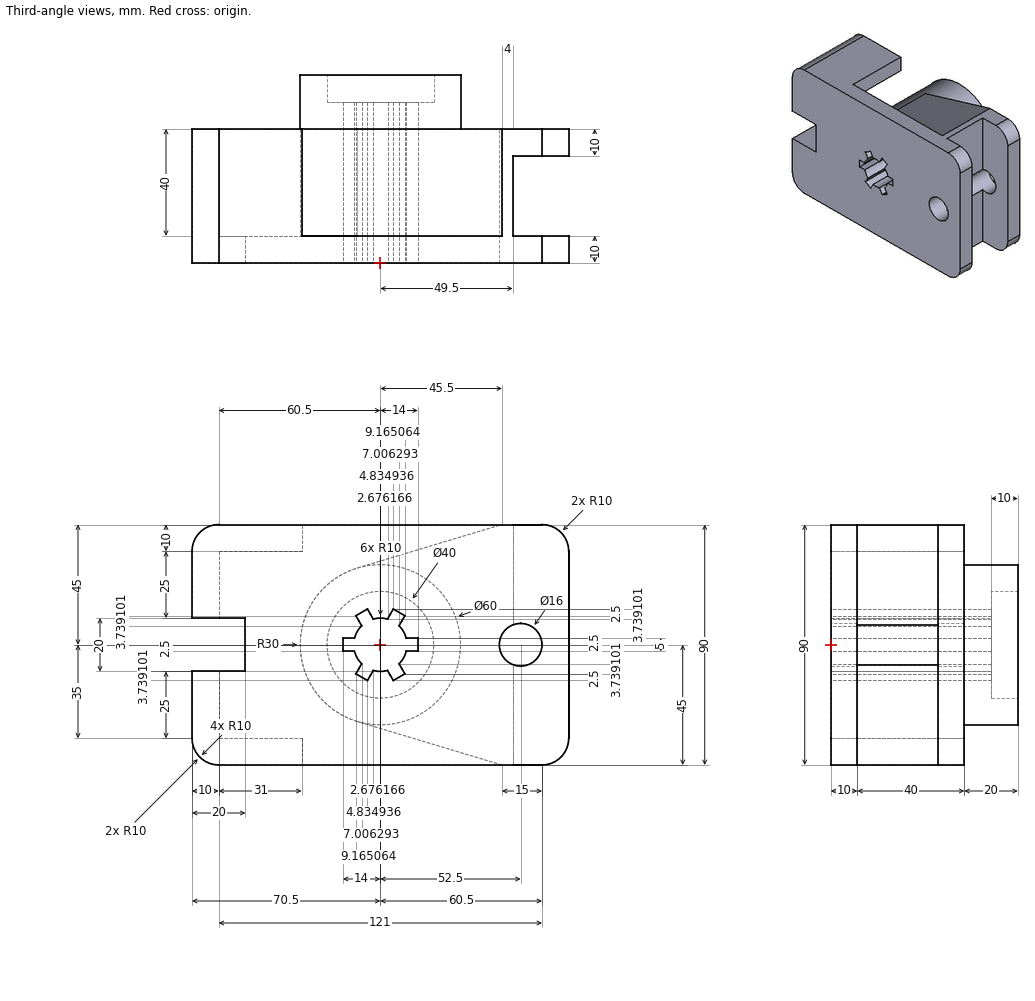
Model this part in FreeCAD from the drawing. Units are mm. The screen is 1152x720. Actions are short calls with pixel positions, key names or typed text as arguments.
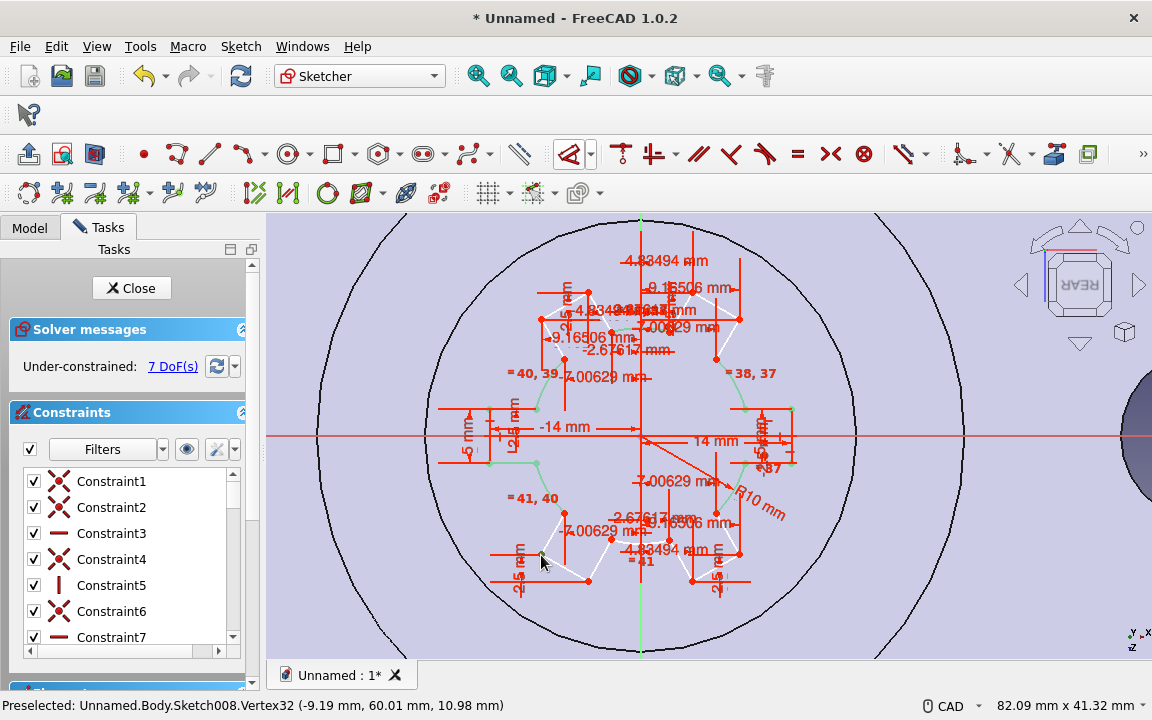
click(590, 154)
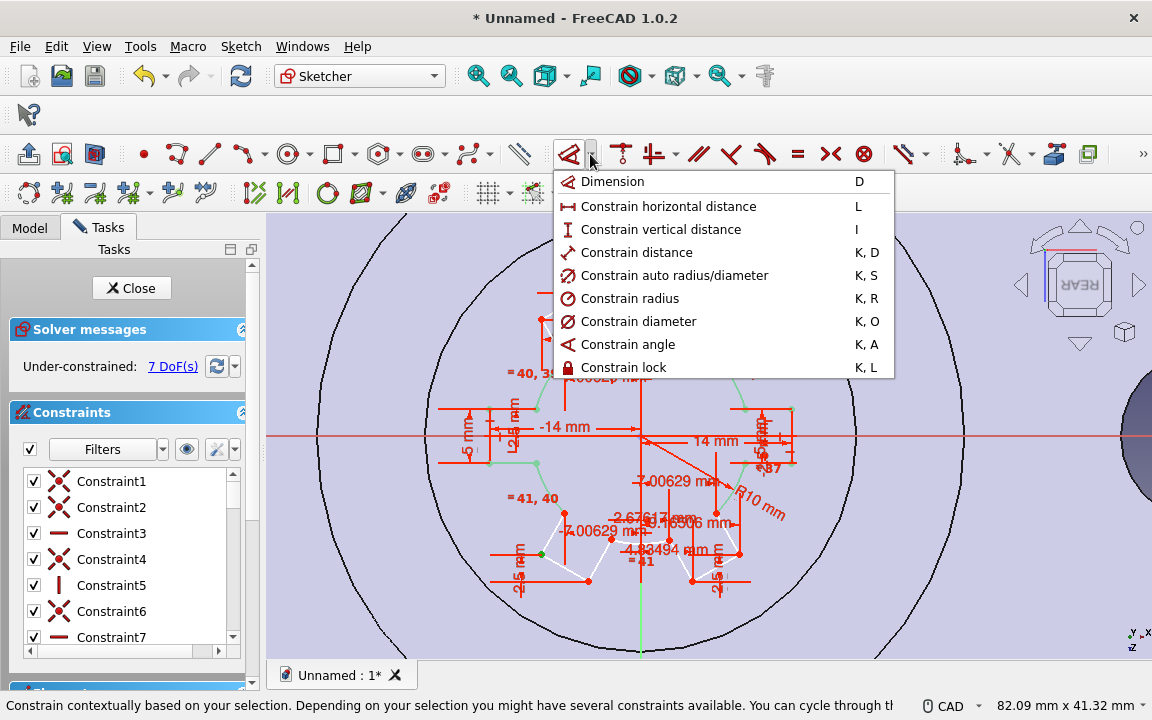
click(724, 206)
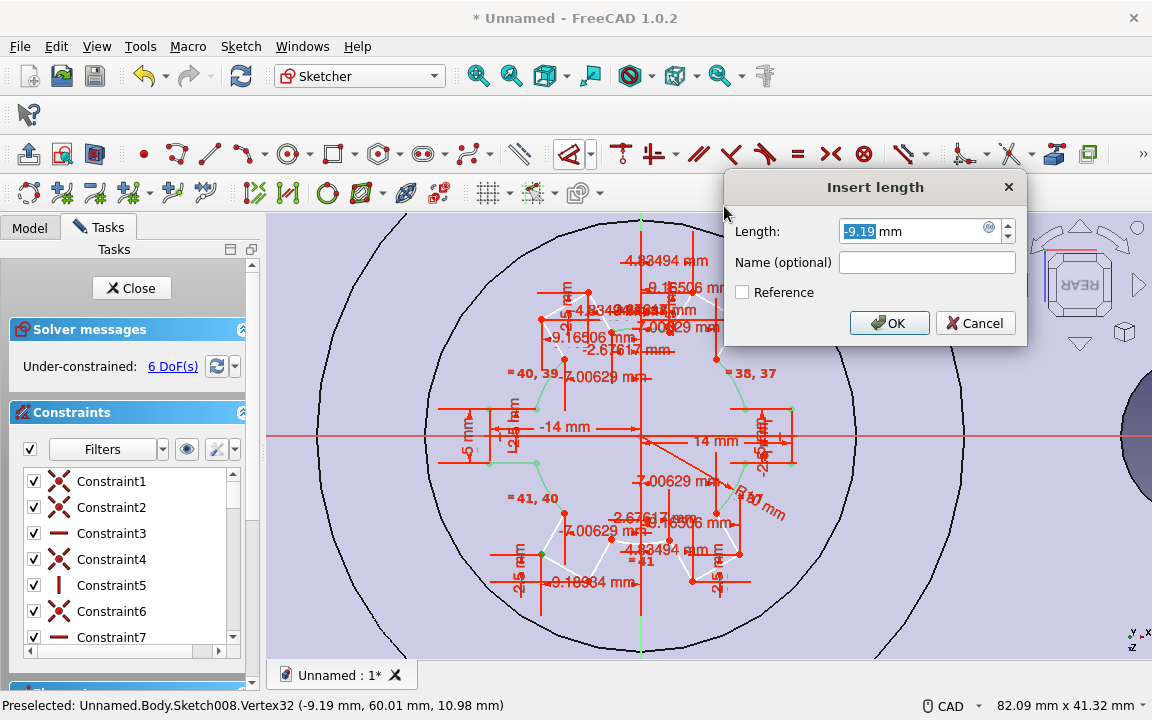
text(-9.165064)
key(Return)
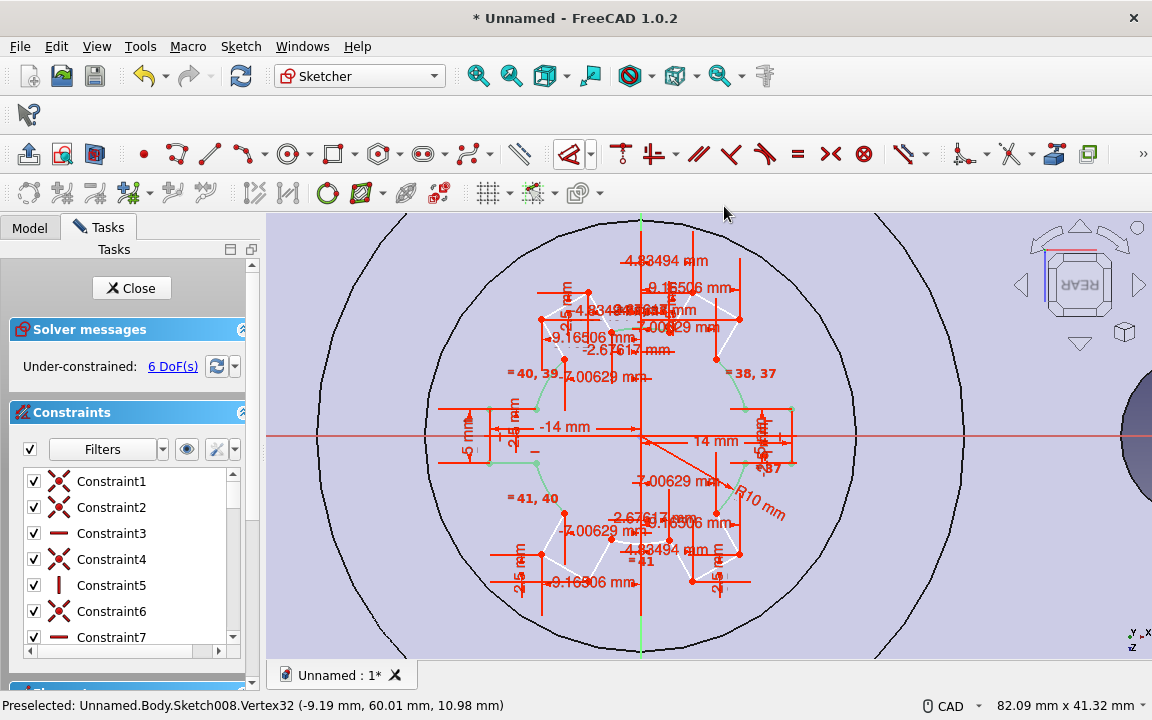
click(588, 582)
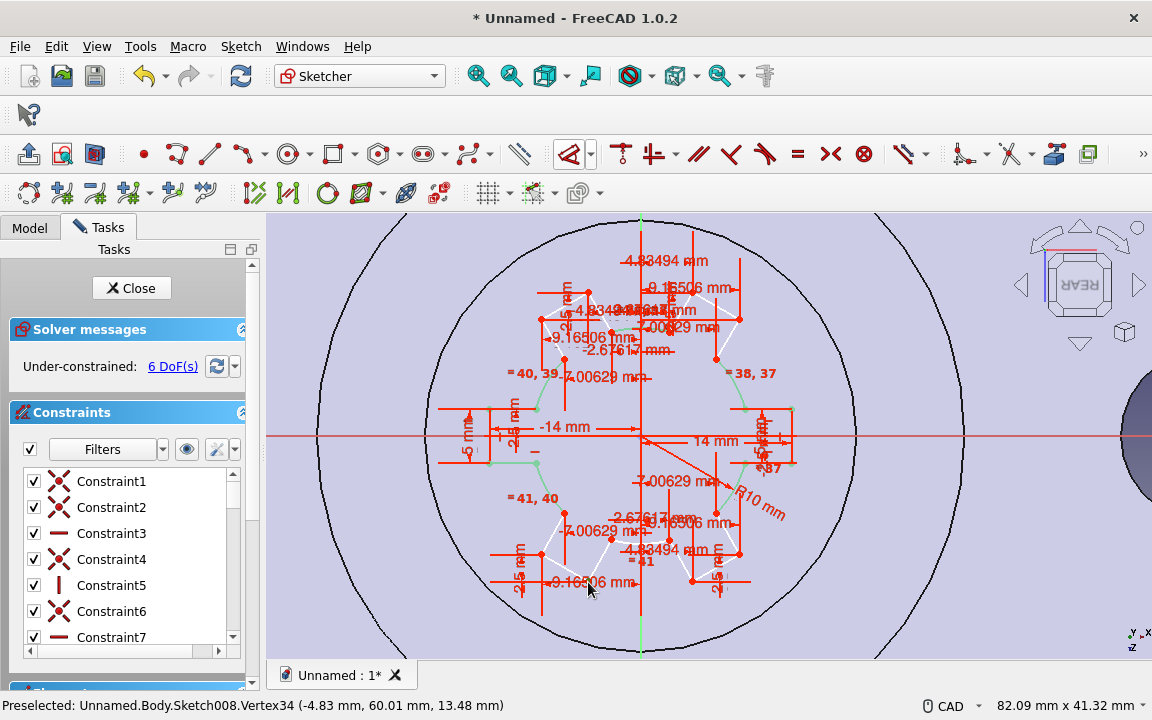
key(l)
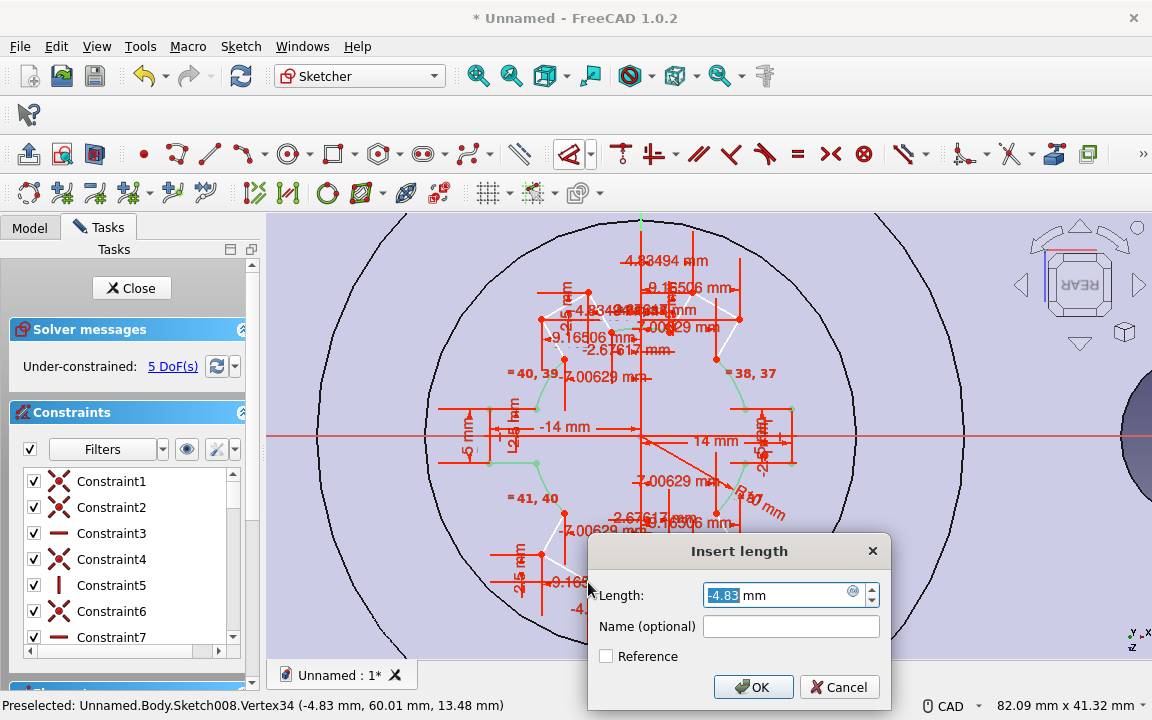
text(-4.834936)
key(Return)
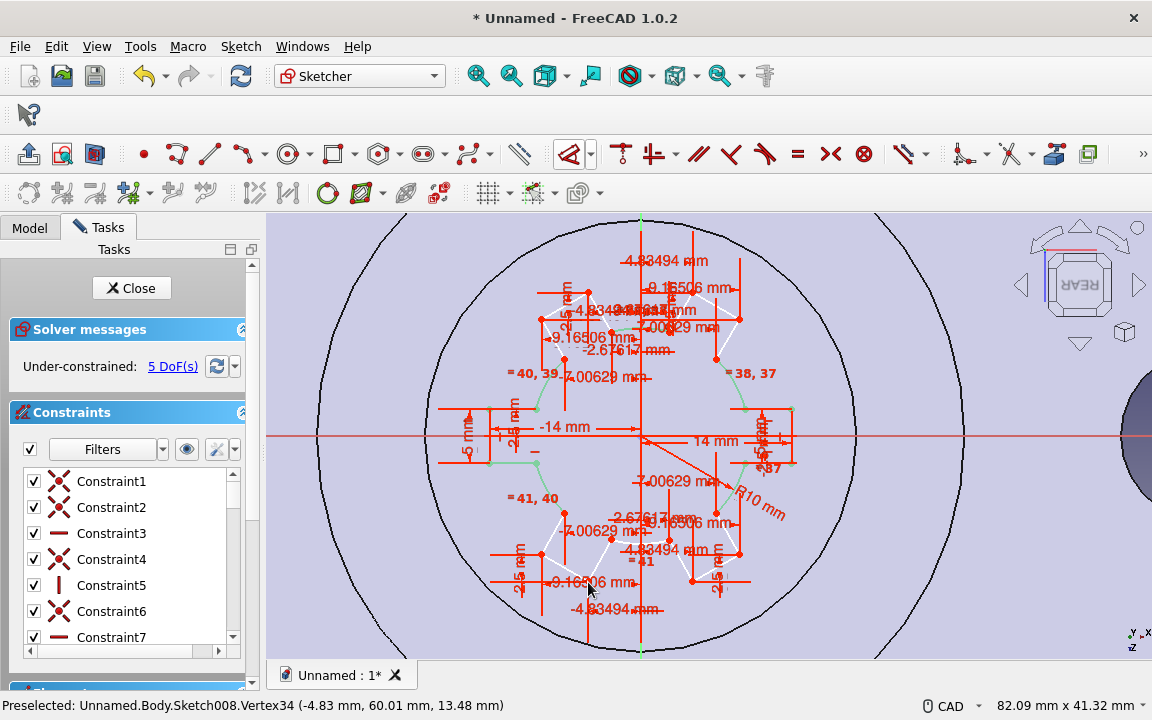
scroll(611, 540, up, 2)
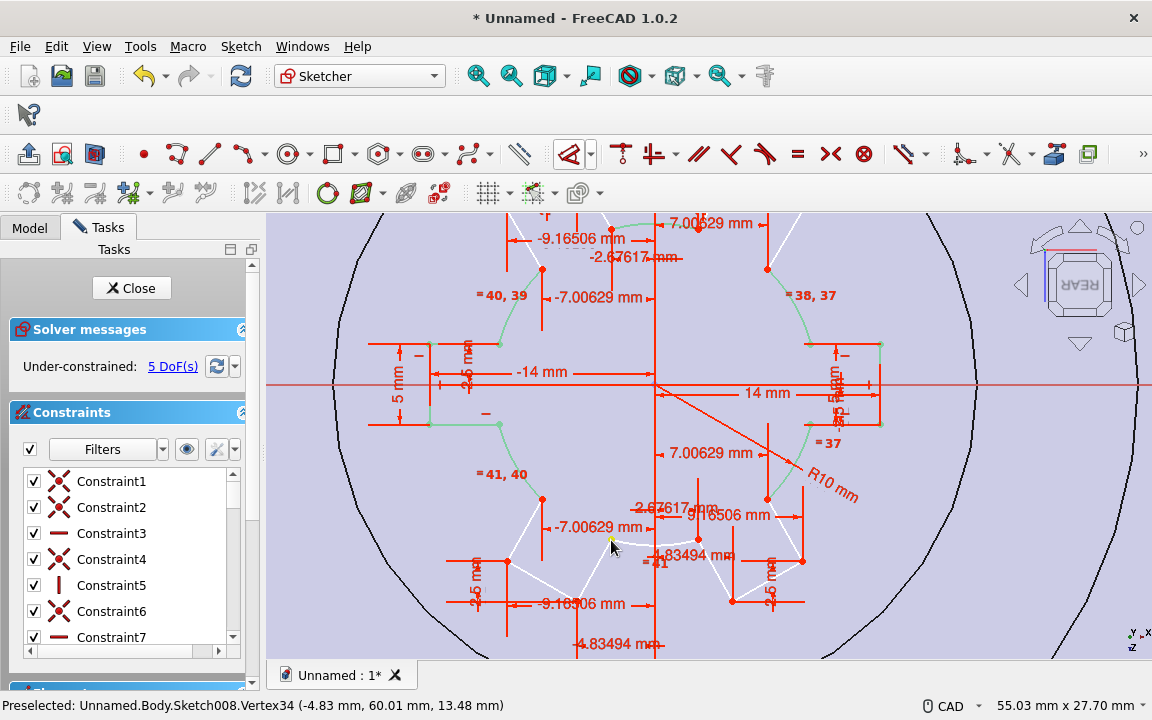
click(611, 540)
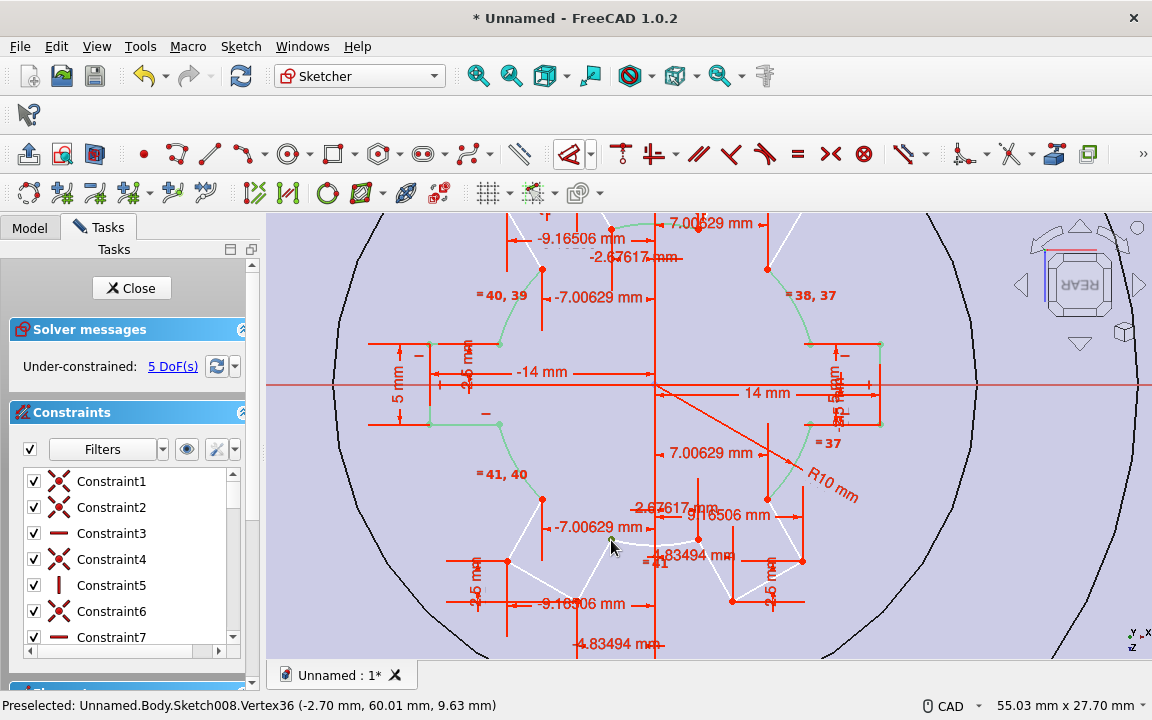
key(l)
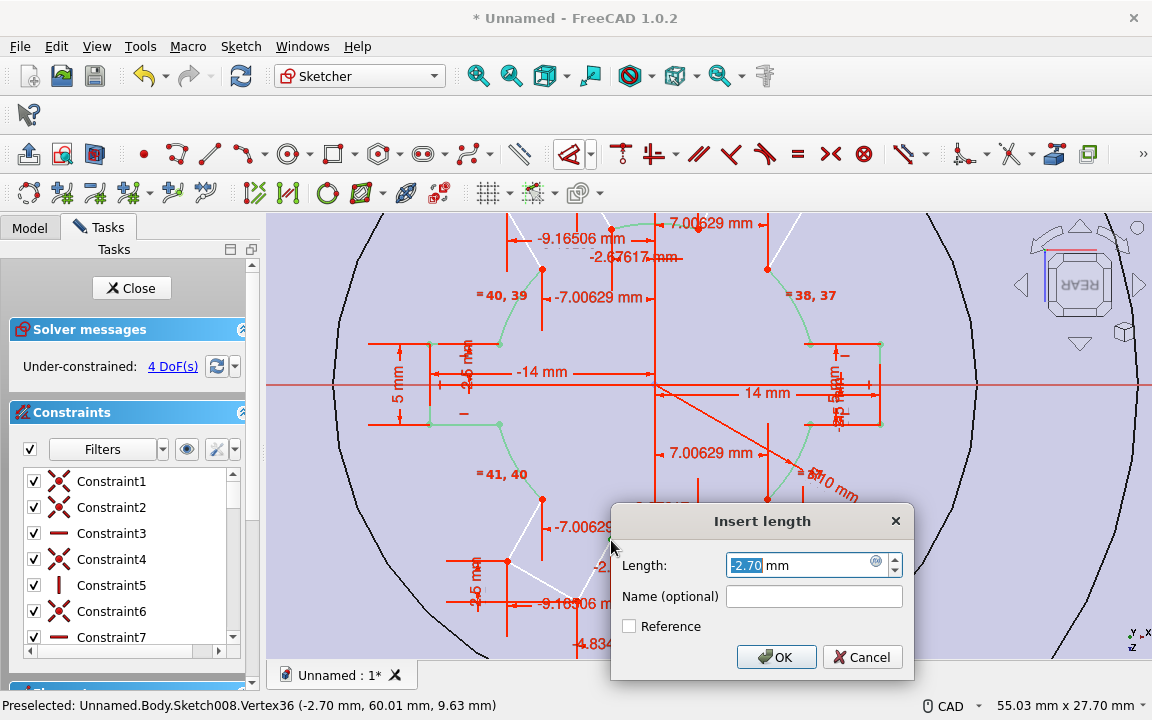
text(-2.676166)
key(Return)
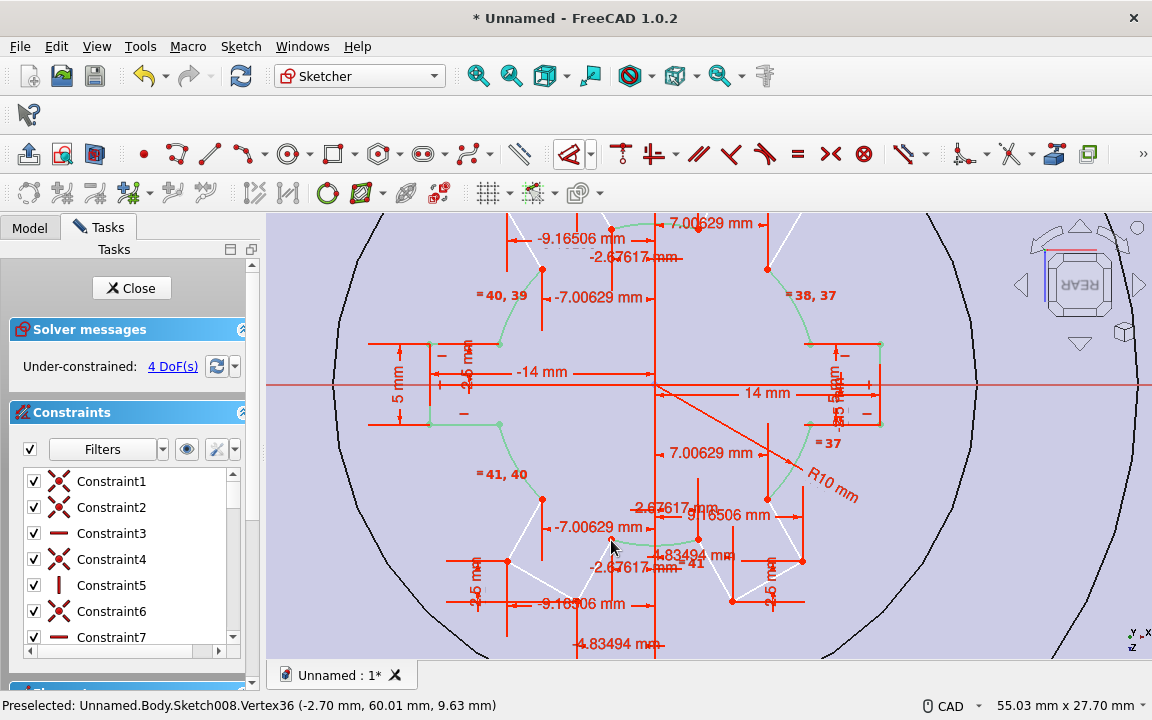
click(722, 583)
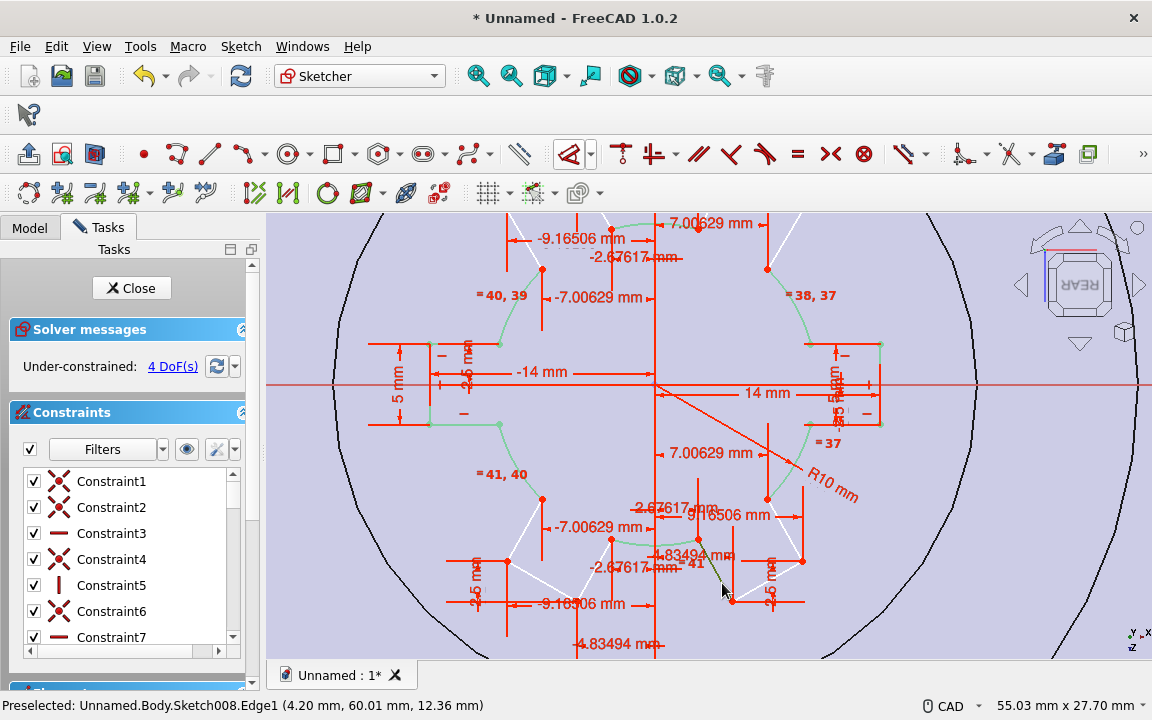
key(i)